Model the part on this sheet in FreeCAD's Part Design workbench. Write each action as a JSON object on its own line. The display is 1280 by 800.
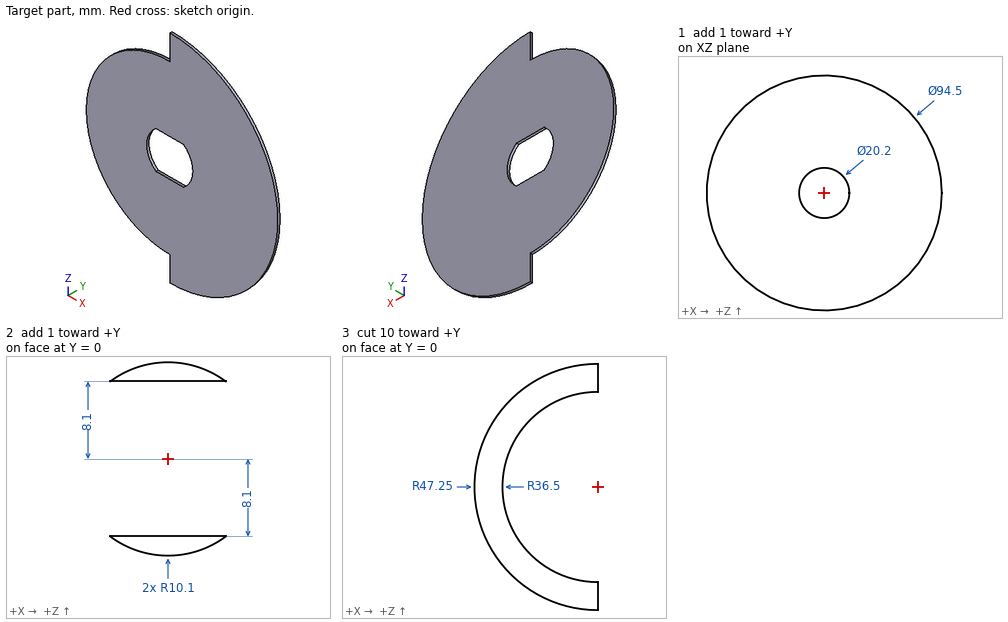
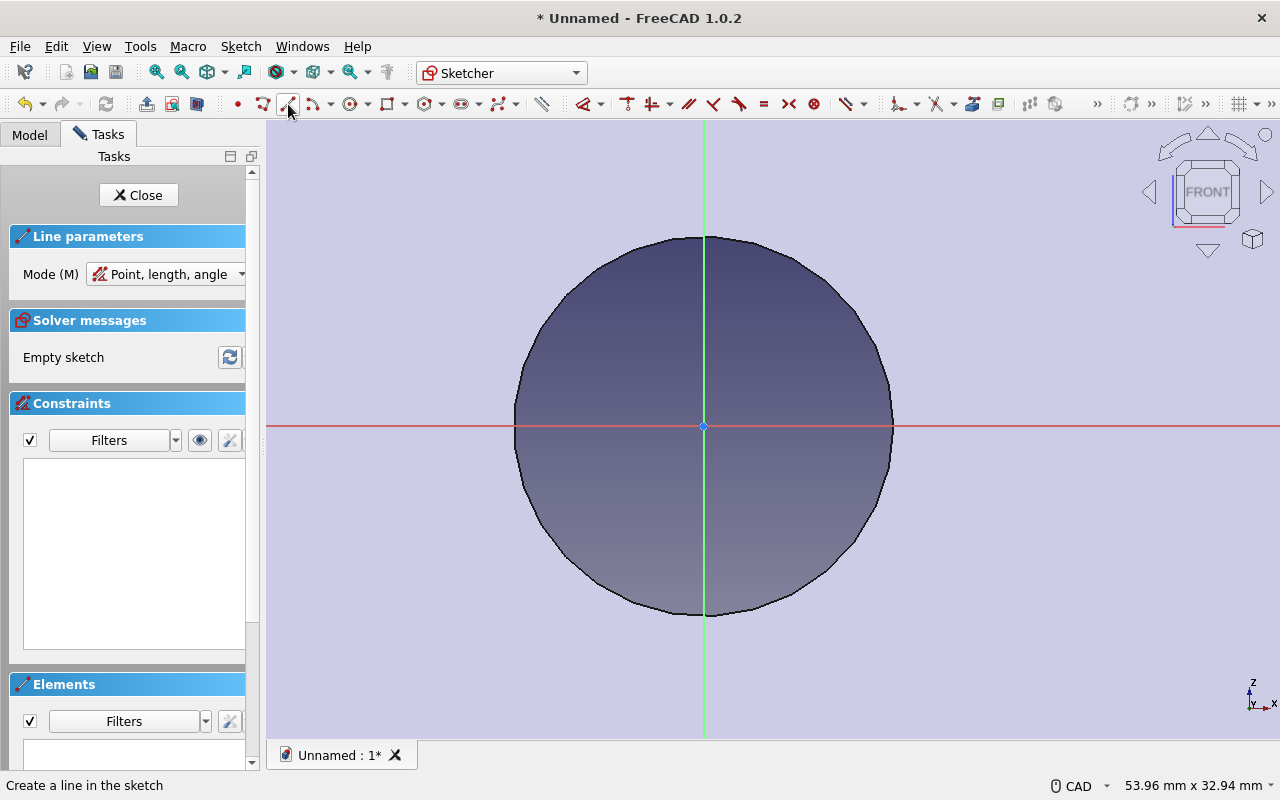
{"action": "left_click", "coordinate": [817, 579]}
{"action": "left_click", "coordinate": [590, 579]}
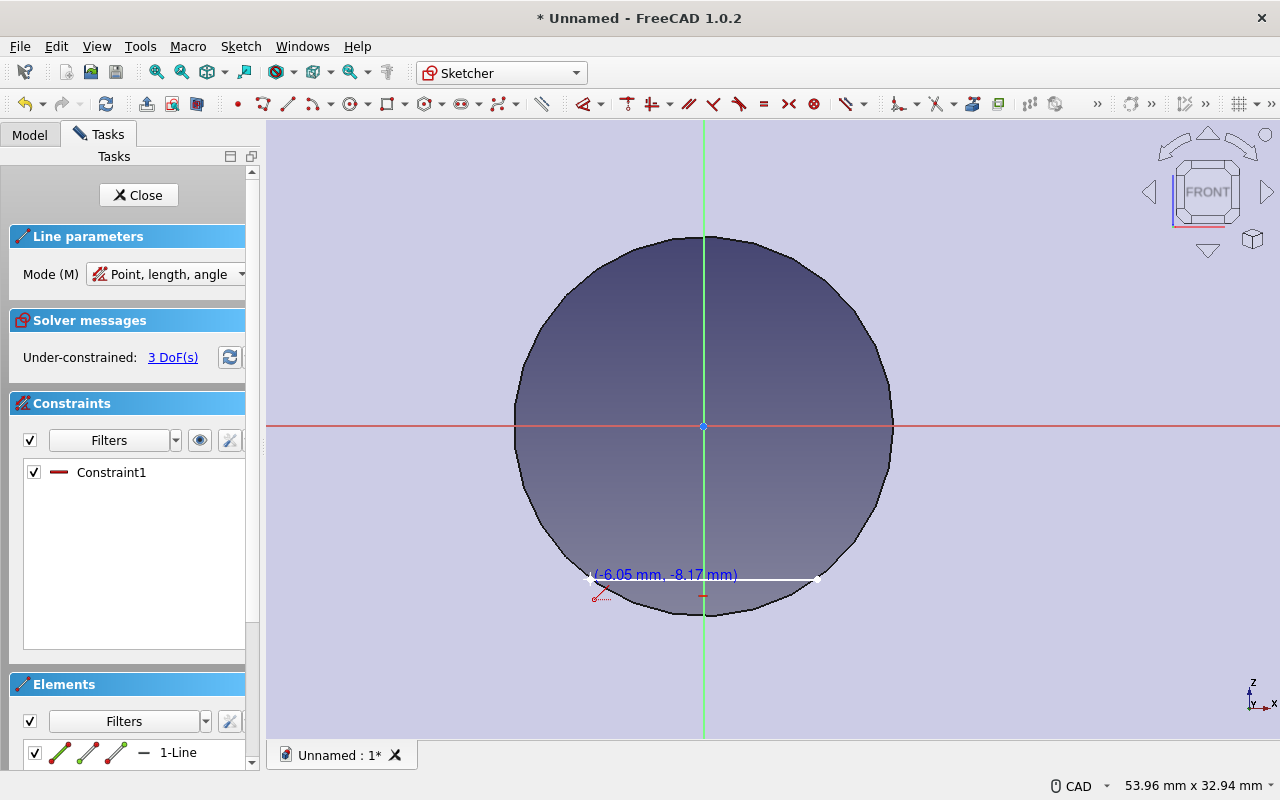
{"action": "left_click", "coordinate": [330, 104]}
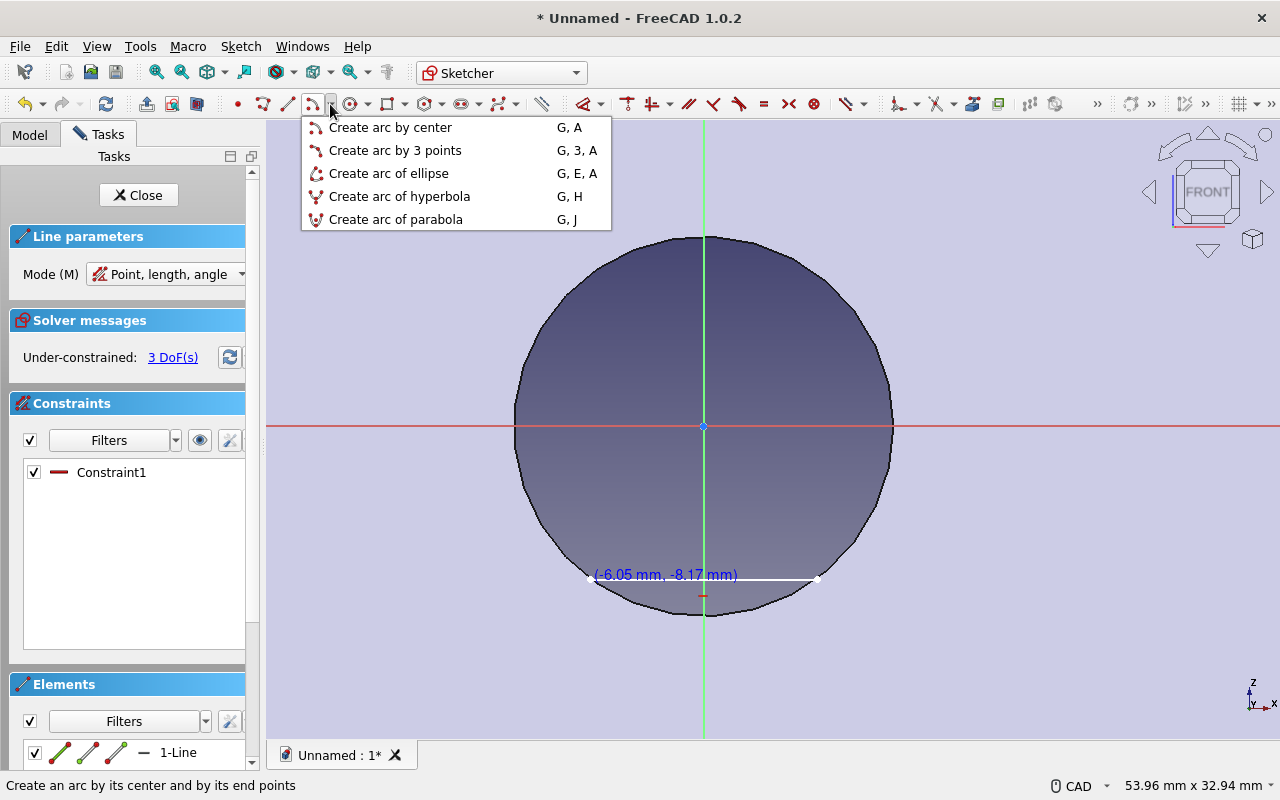
{"action": "left_click", "coordinate": [456, 150]}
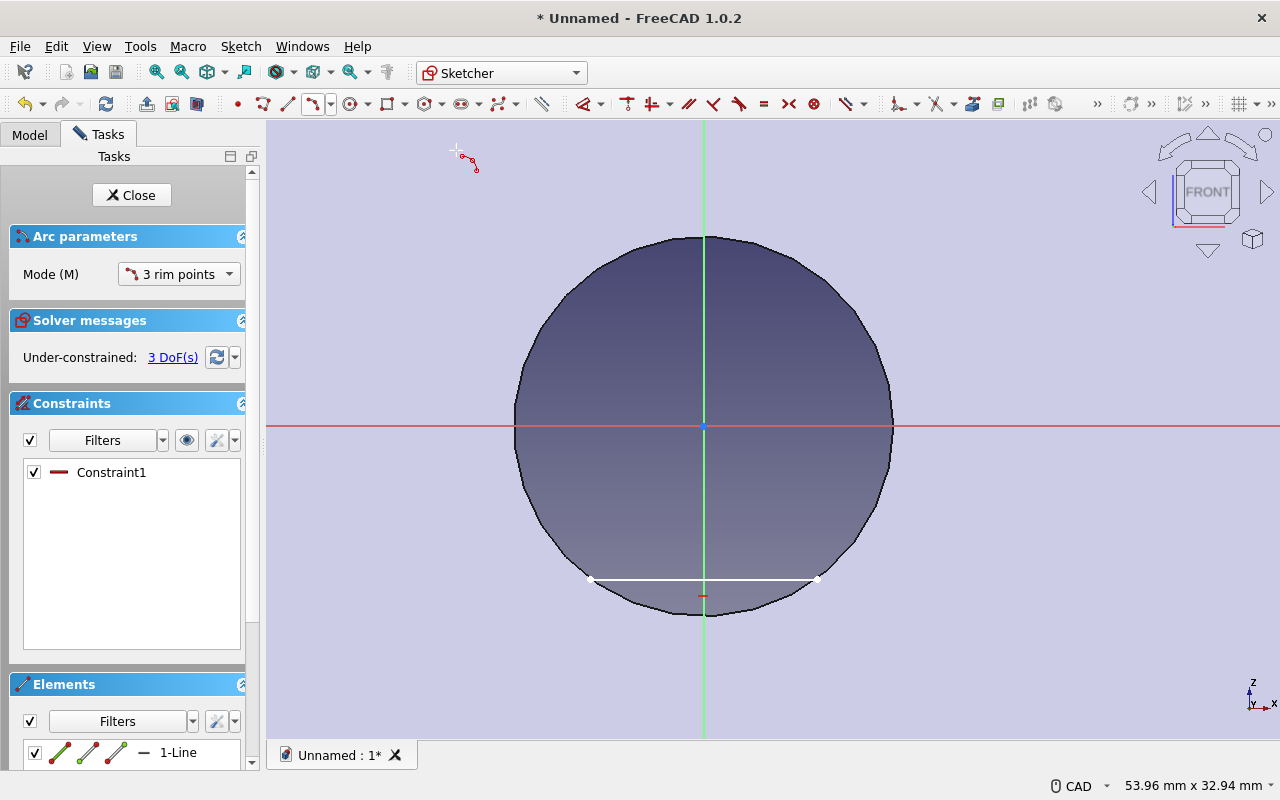
{"action": "left_click", "coordinate": [590, 580]}
{"action": "left_click", "coordinate": [817, 580]}
{"action": "left_click", "coordinate": [679, 615]}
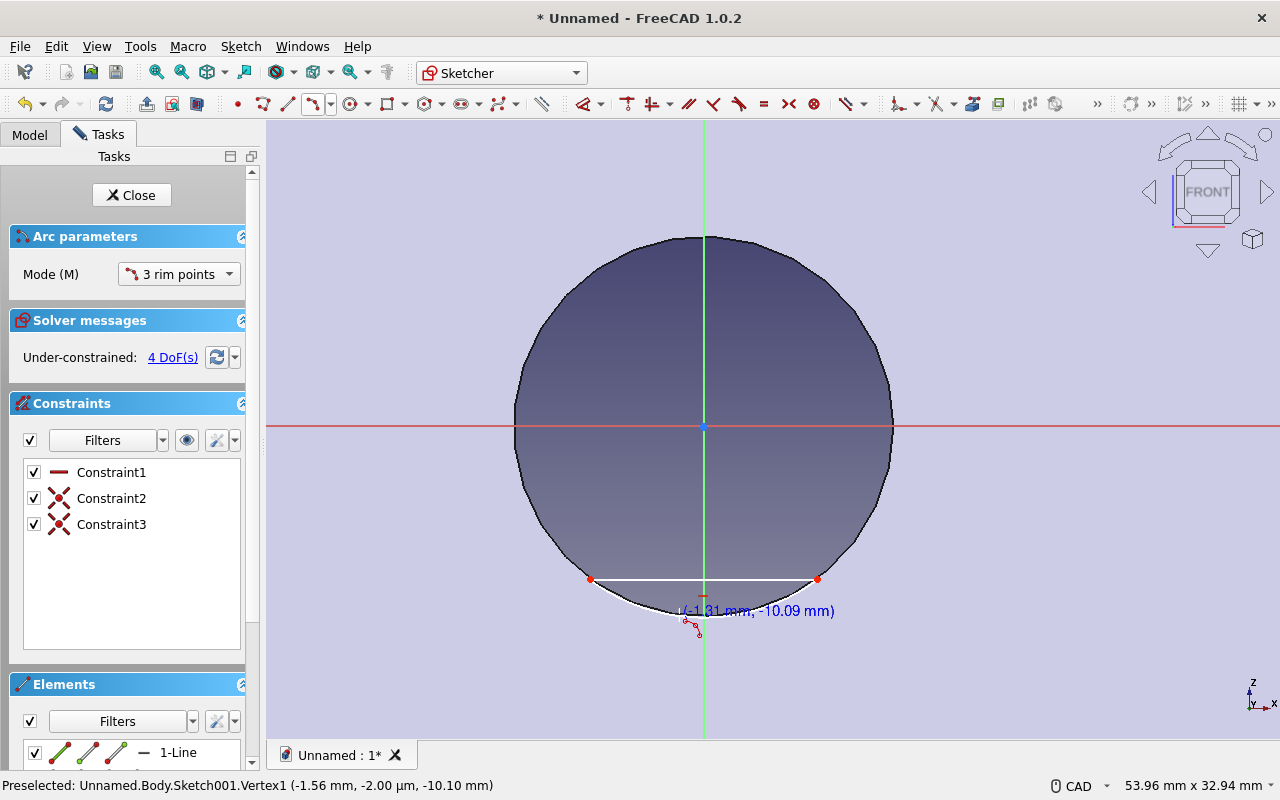
{"action": "left_click", "coordinate": [288, 104]}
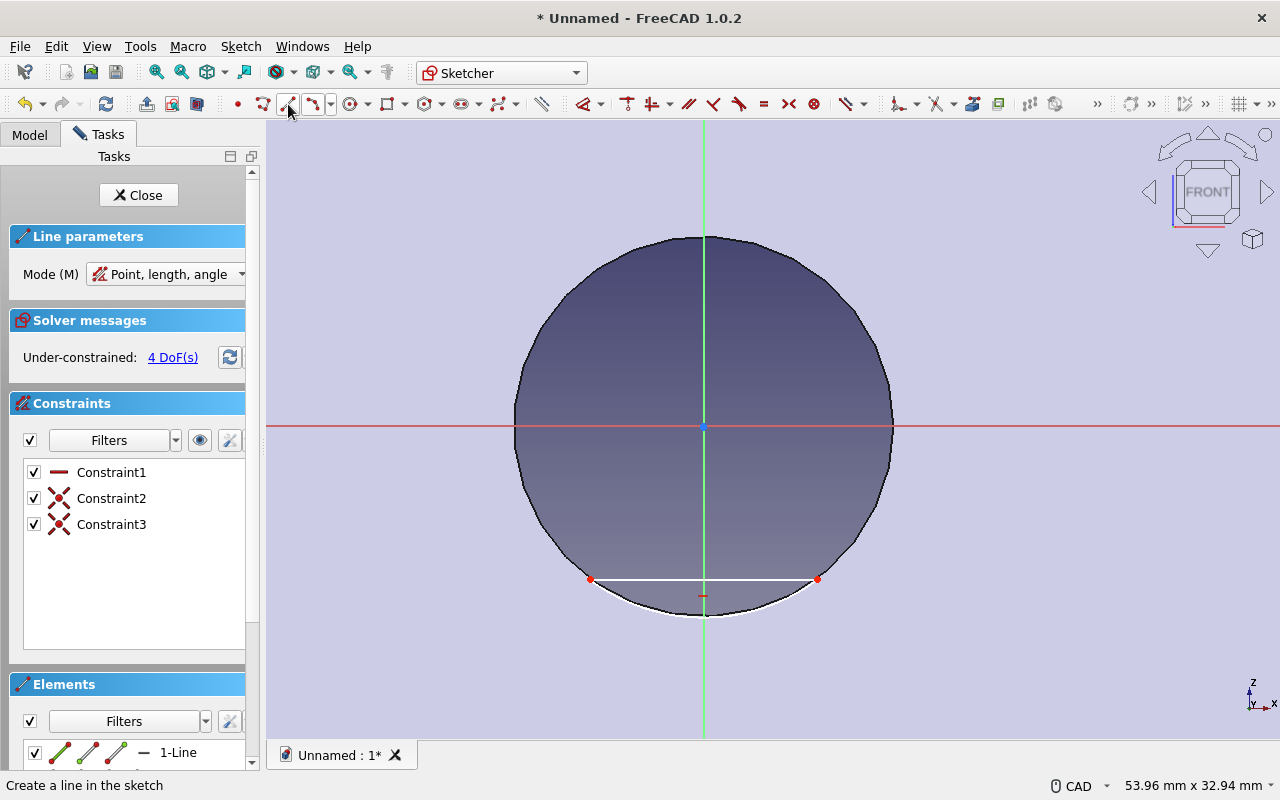
{"action": "left_click", "coordinate": [590, 274]}
{"action": "left_click", "coordinate": [817, 274]}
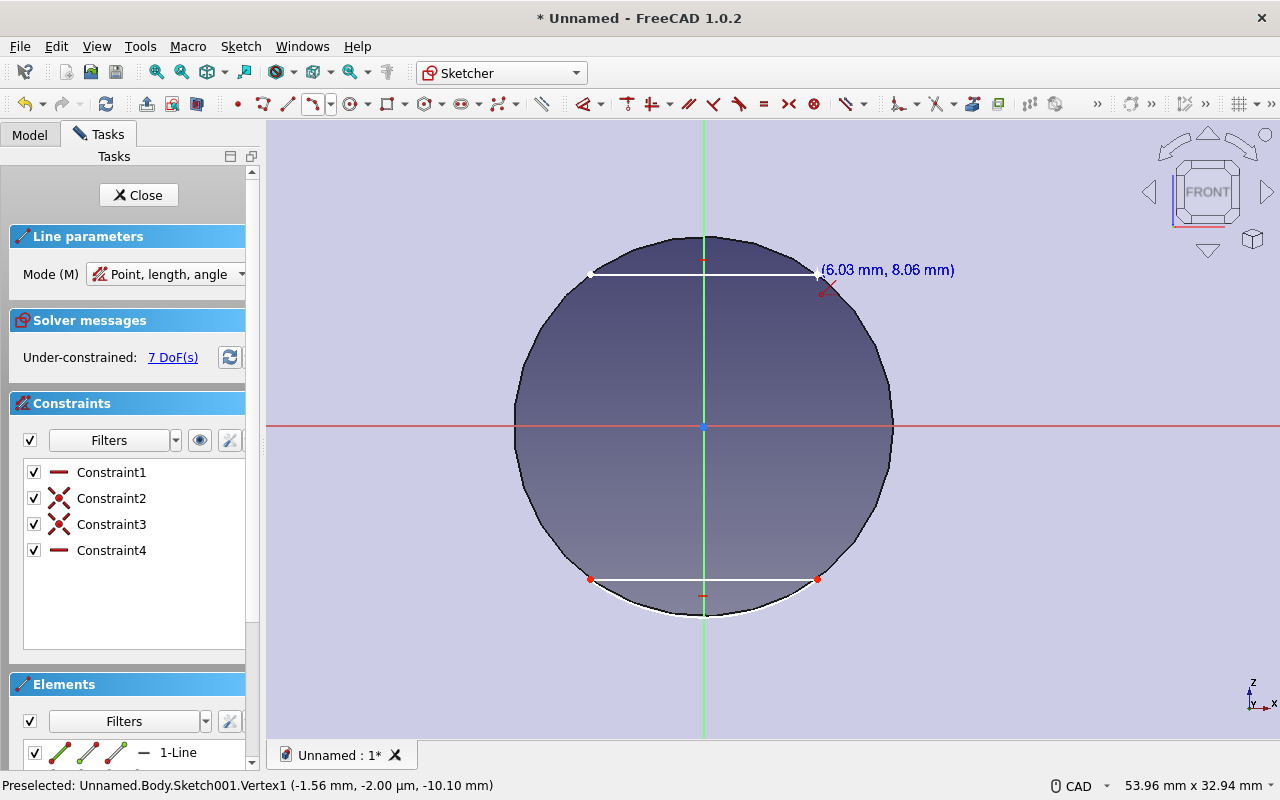
{"action": "left_click", "coordinate": [312, 104]}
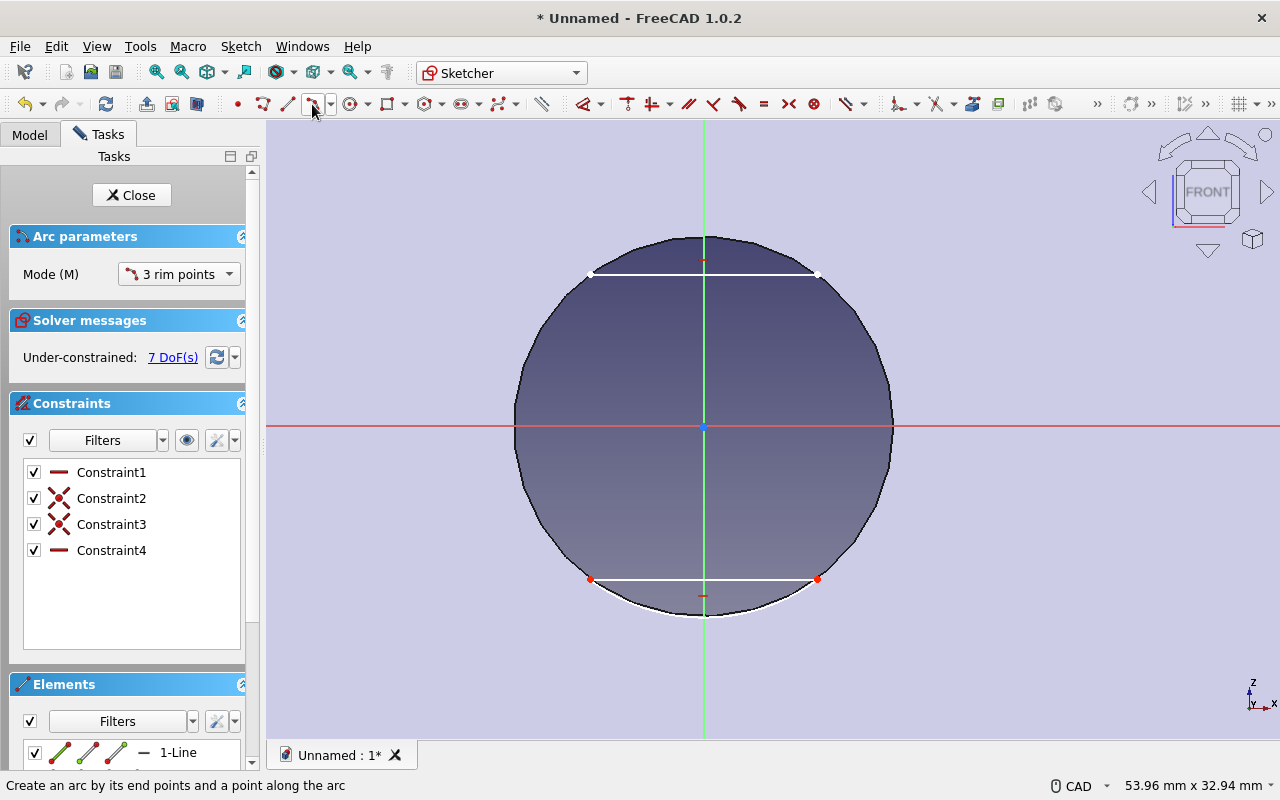
{"action": "left_click", "coordinate": [817, 275]}
{"action": "left_click", "coordinate": [590, 275]}
{"action": "left_click", "coordinate": [728, 238]}
{"action": "key", "text": "Escape"}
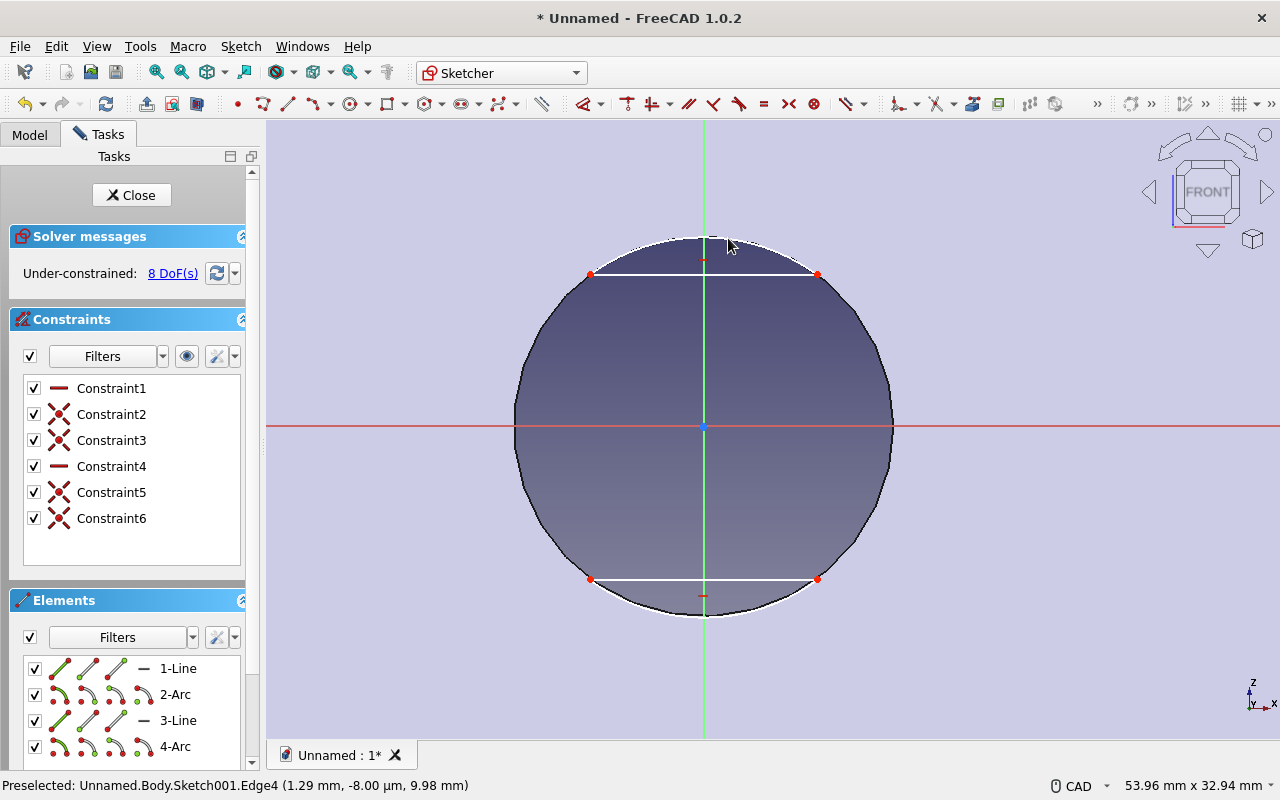
{"action": "left_click", "coordinate": [655, 611]}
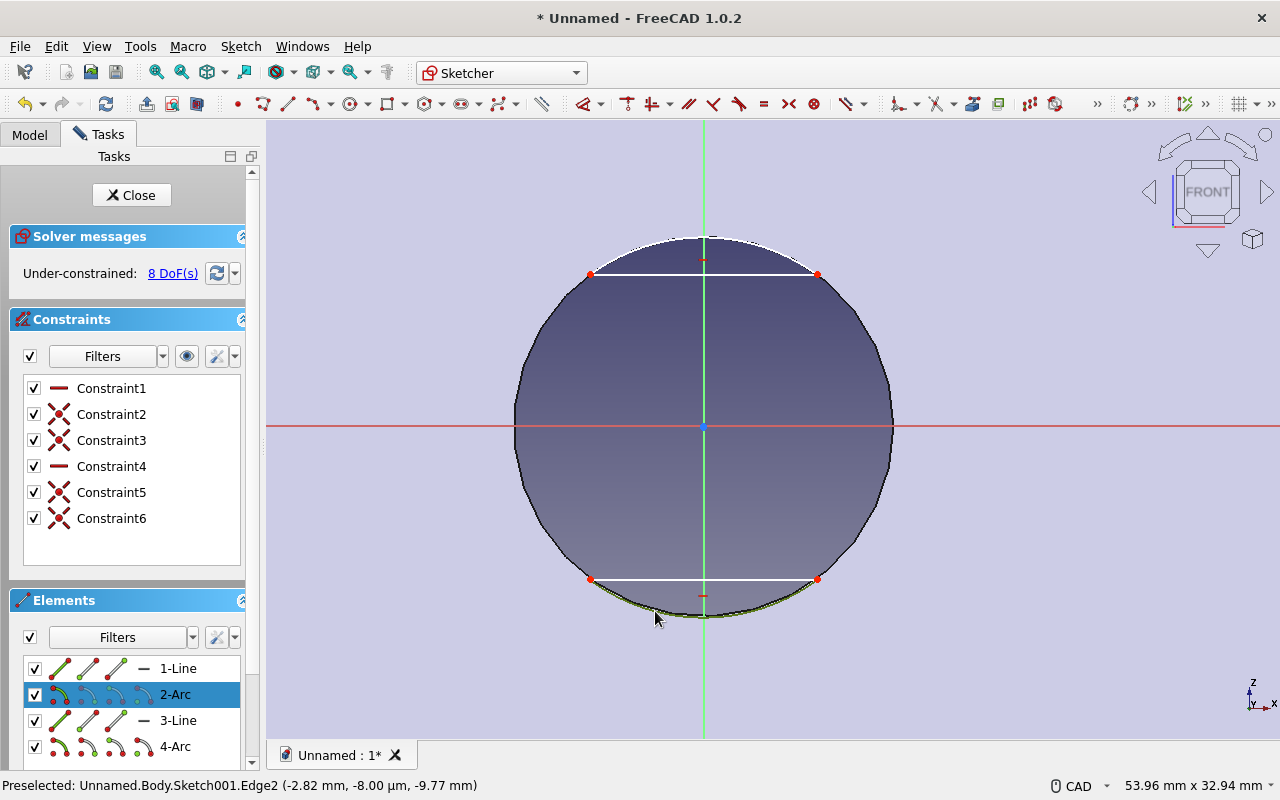
{"action": "left_click", "coordinate": [752, 244]}